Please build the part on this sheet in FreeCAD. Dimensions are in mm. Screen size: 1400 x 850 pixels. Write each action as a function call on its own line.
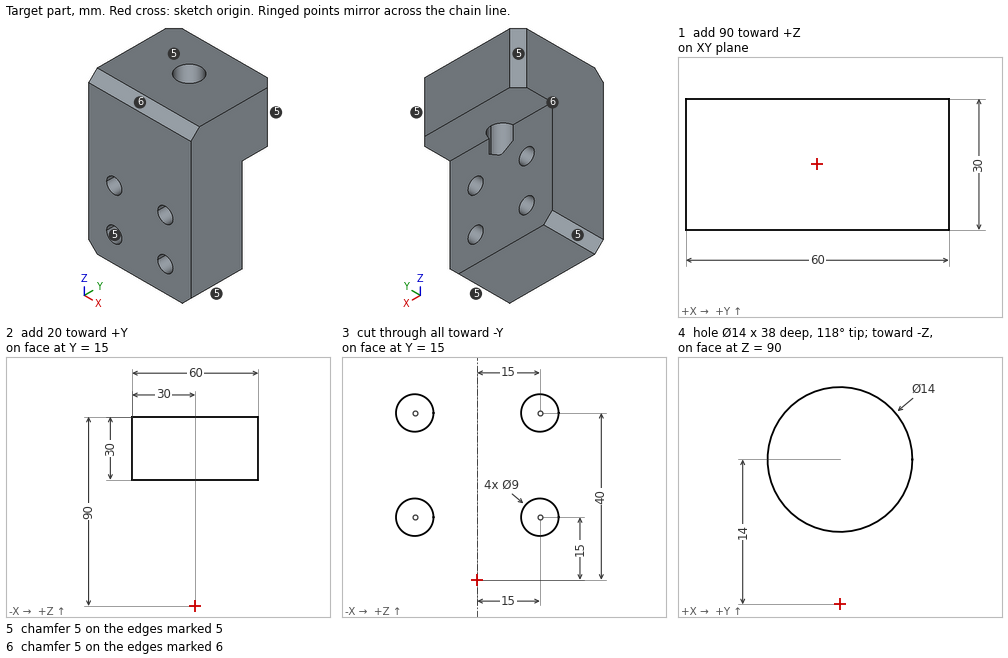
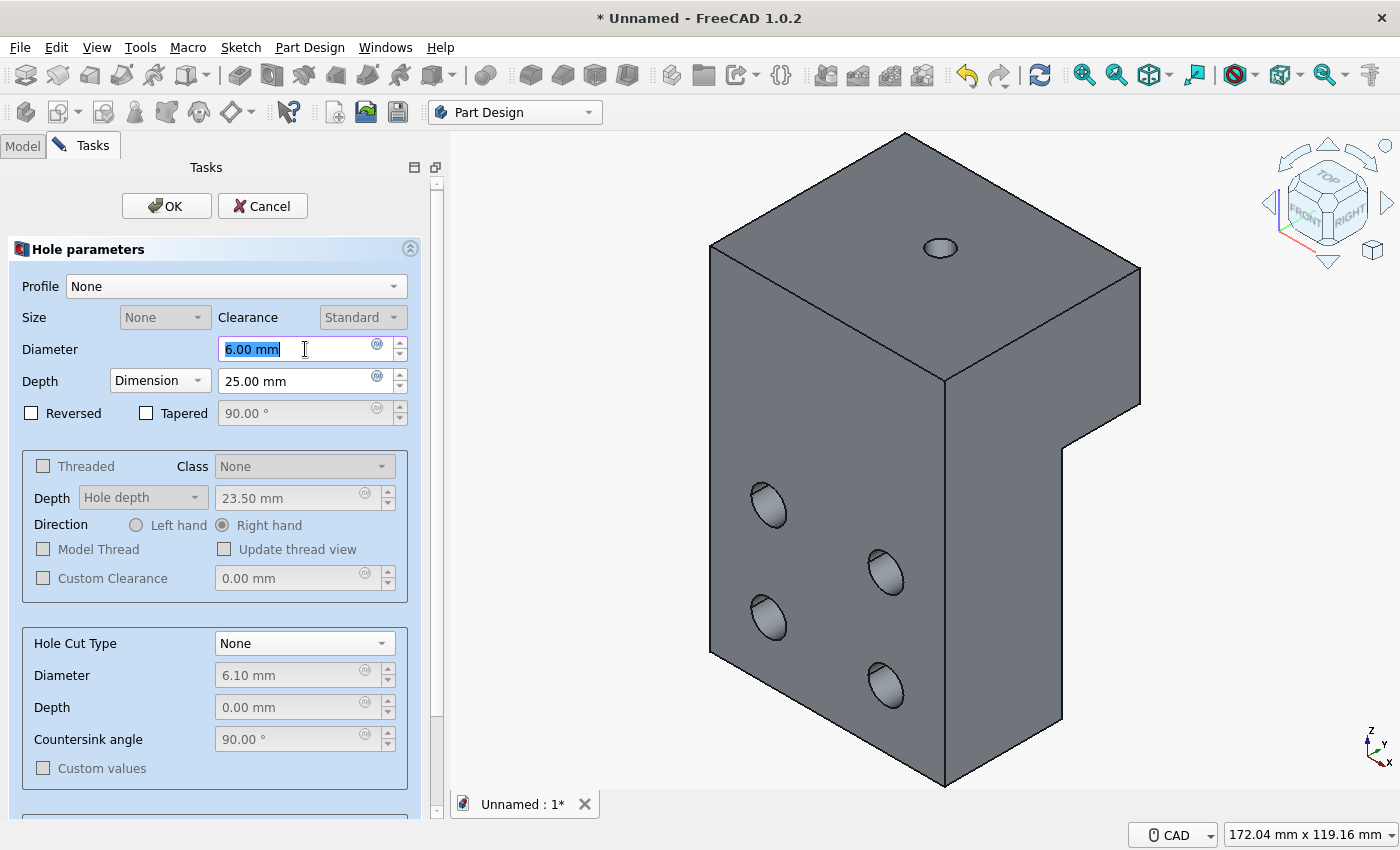
text(14)
key(Tab)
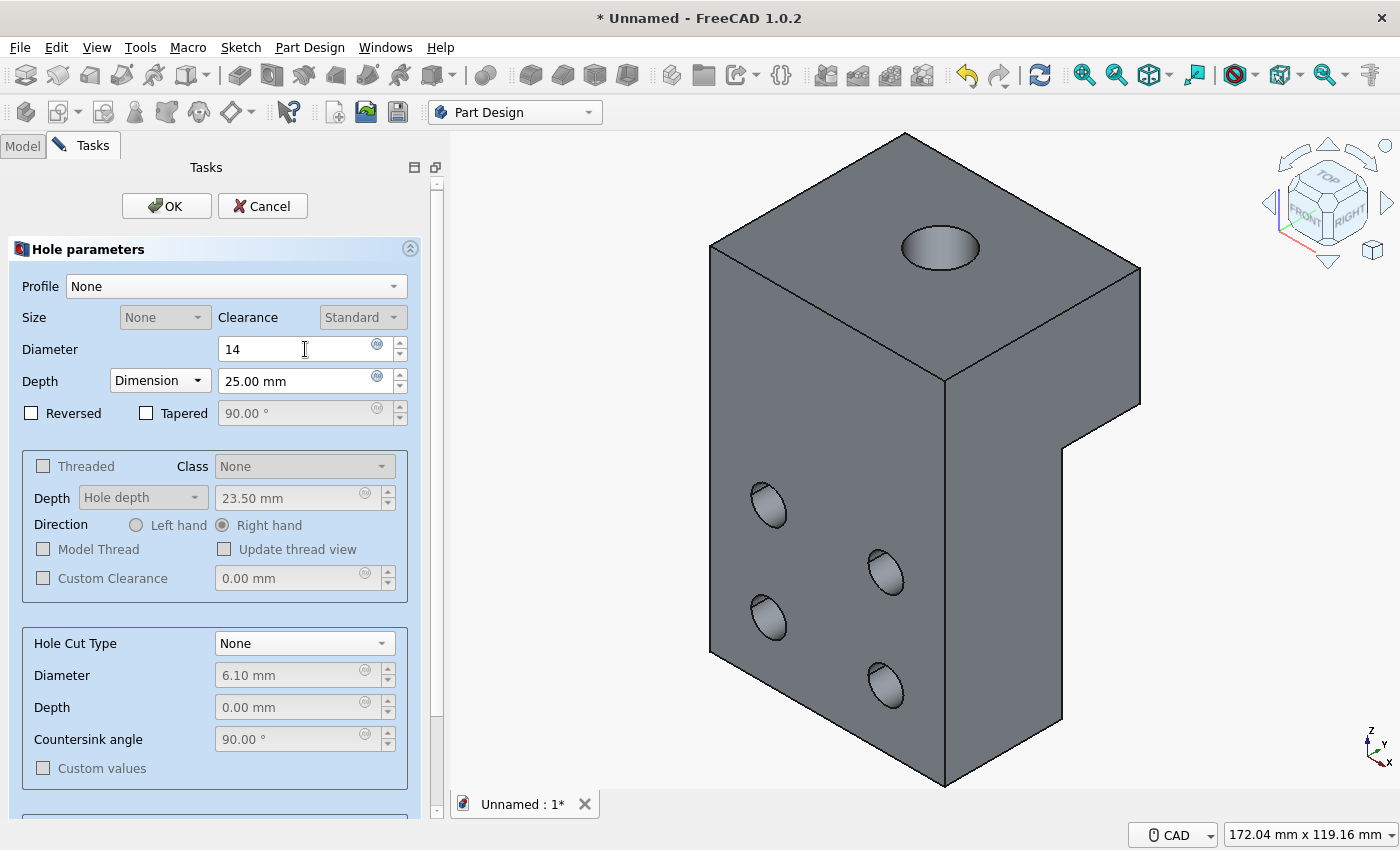
triple_click(305, 381)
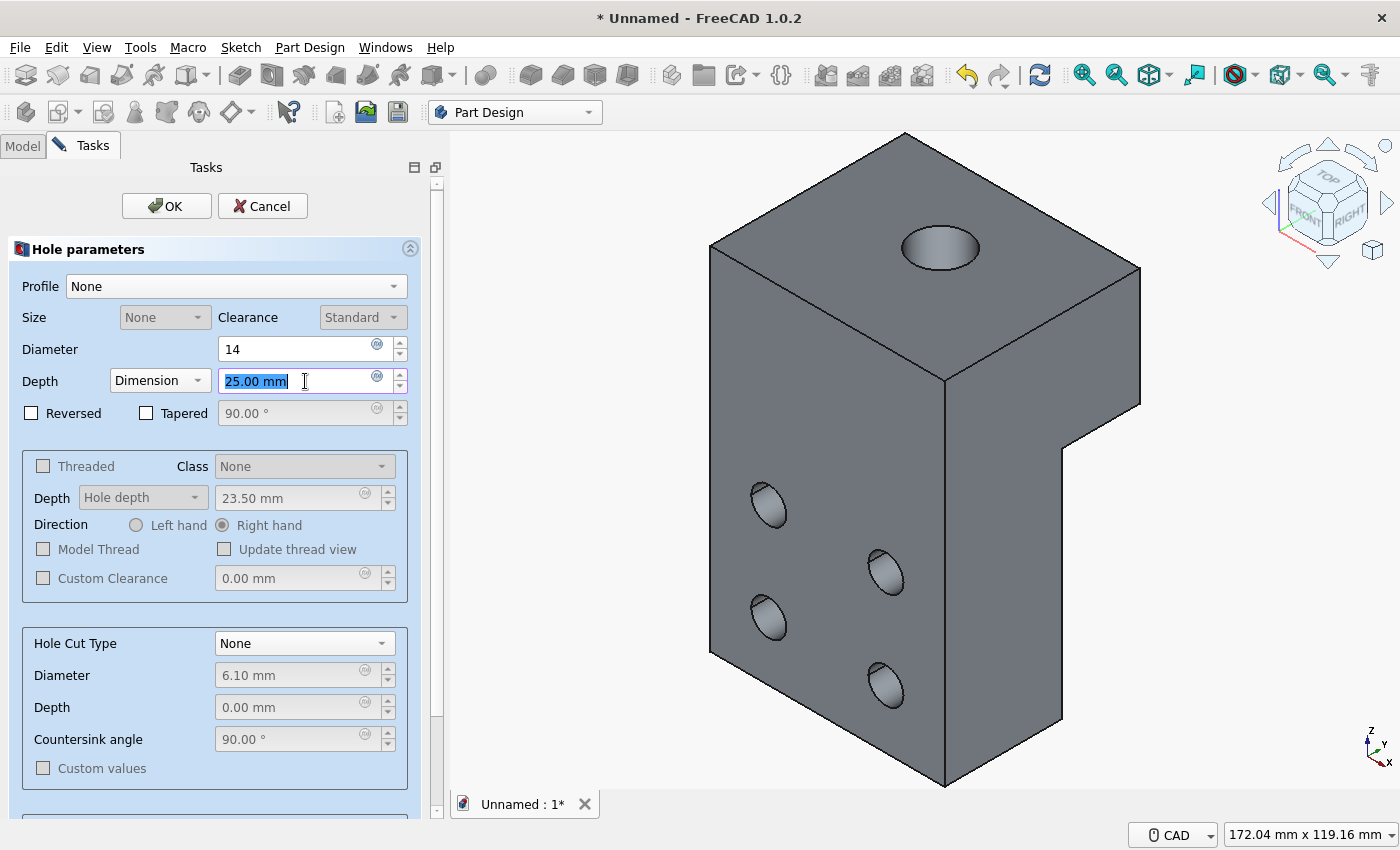
text(38)
key(Tab)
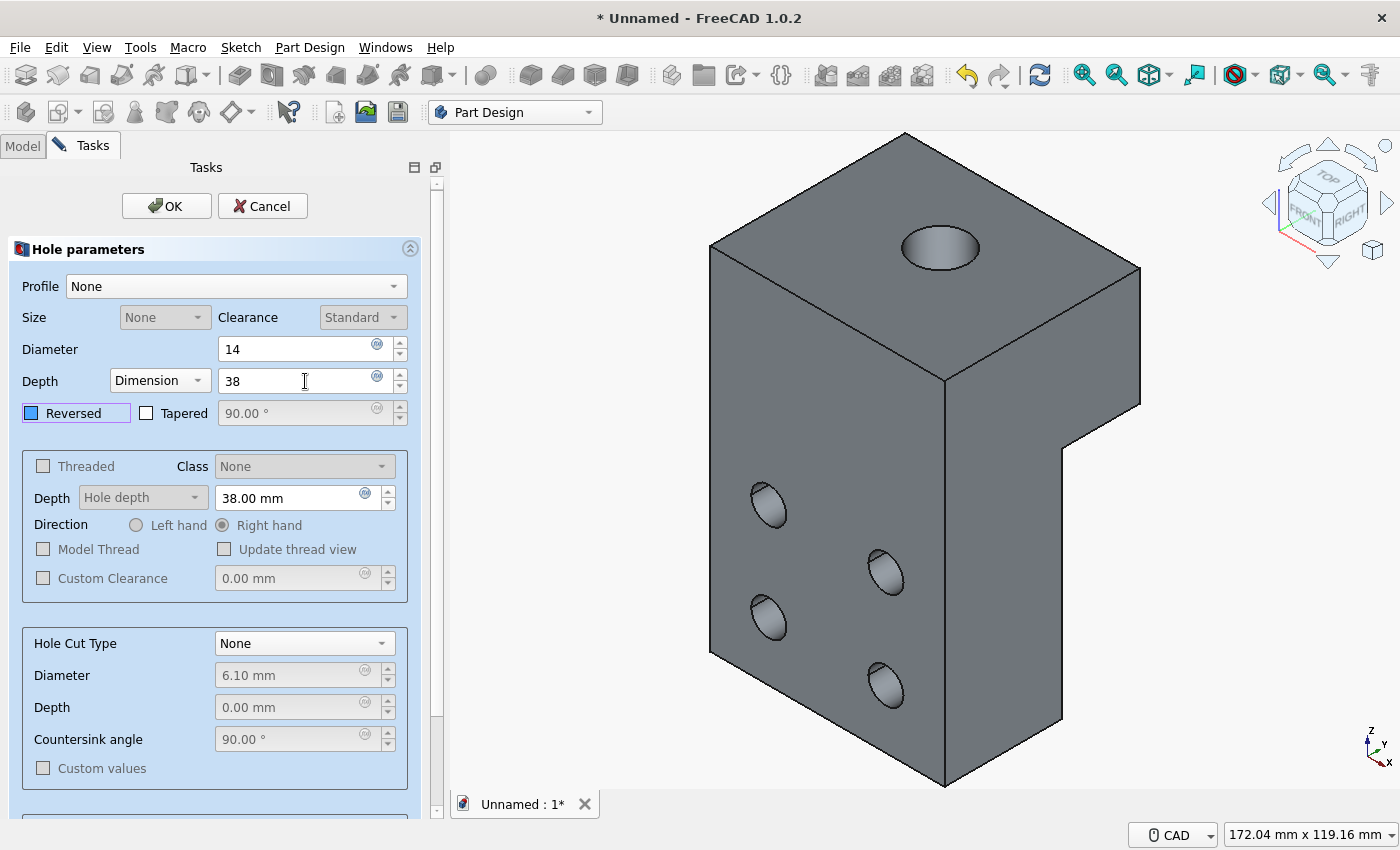
click(167, 206)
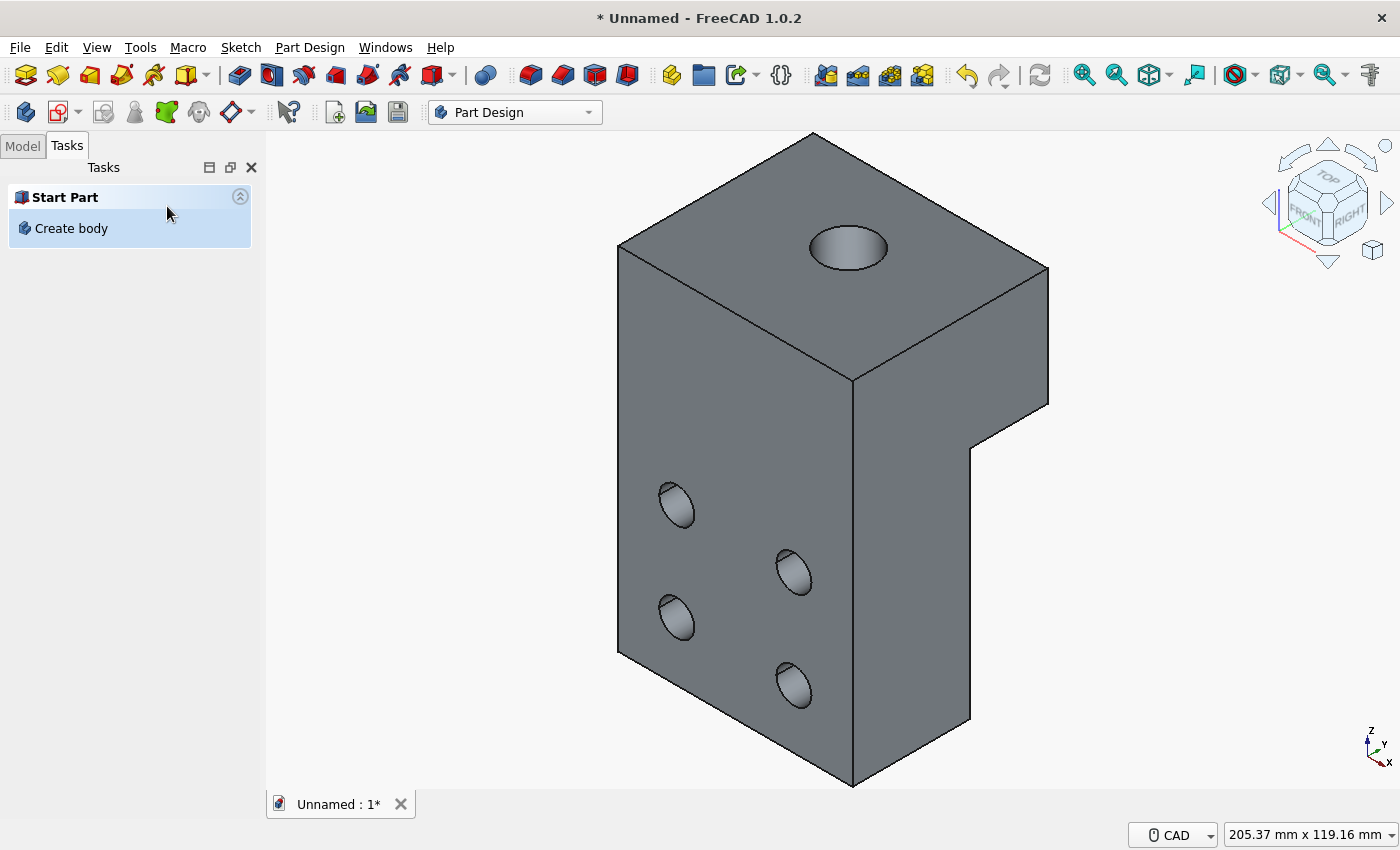
key(2)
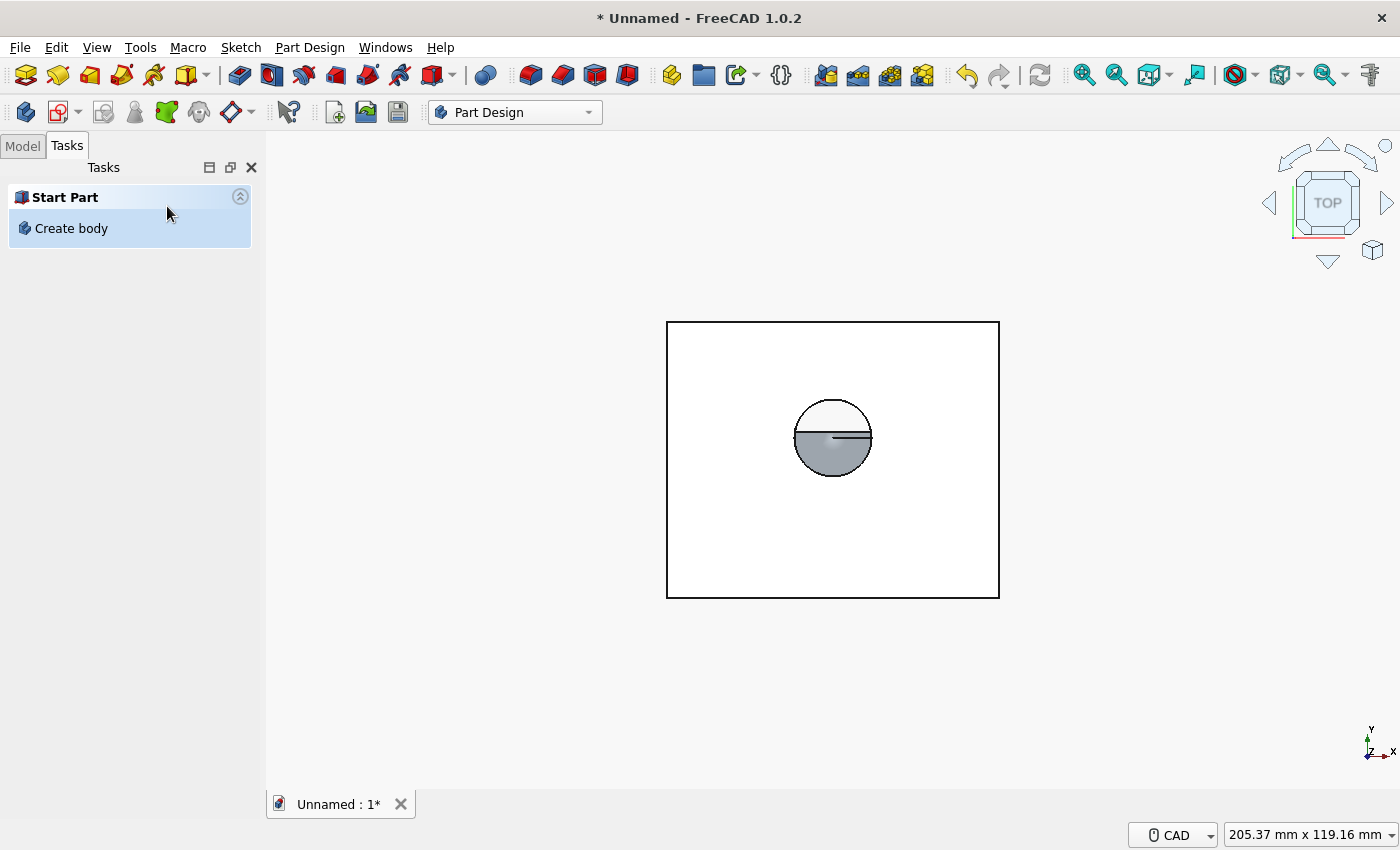
click(1086, 76)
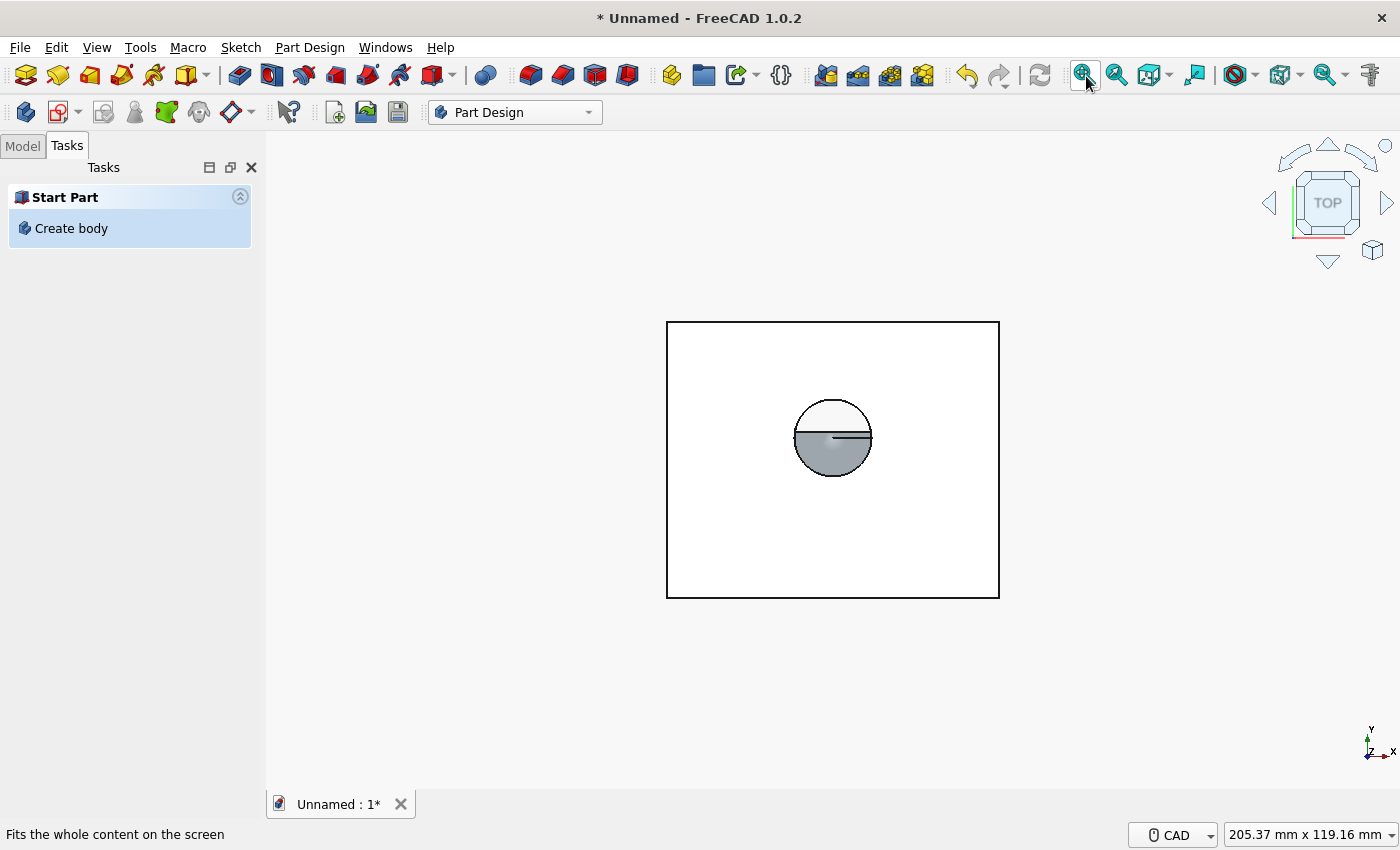
key(0)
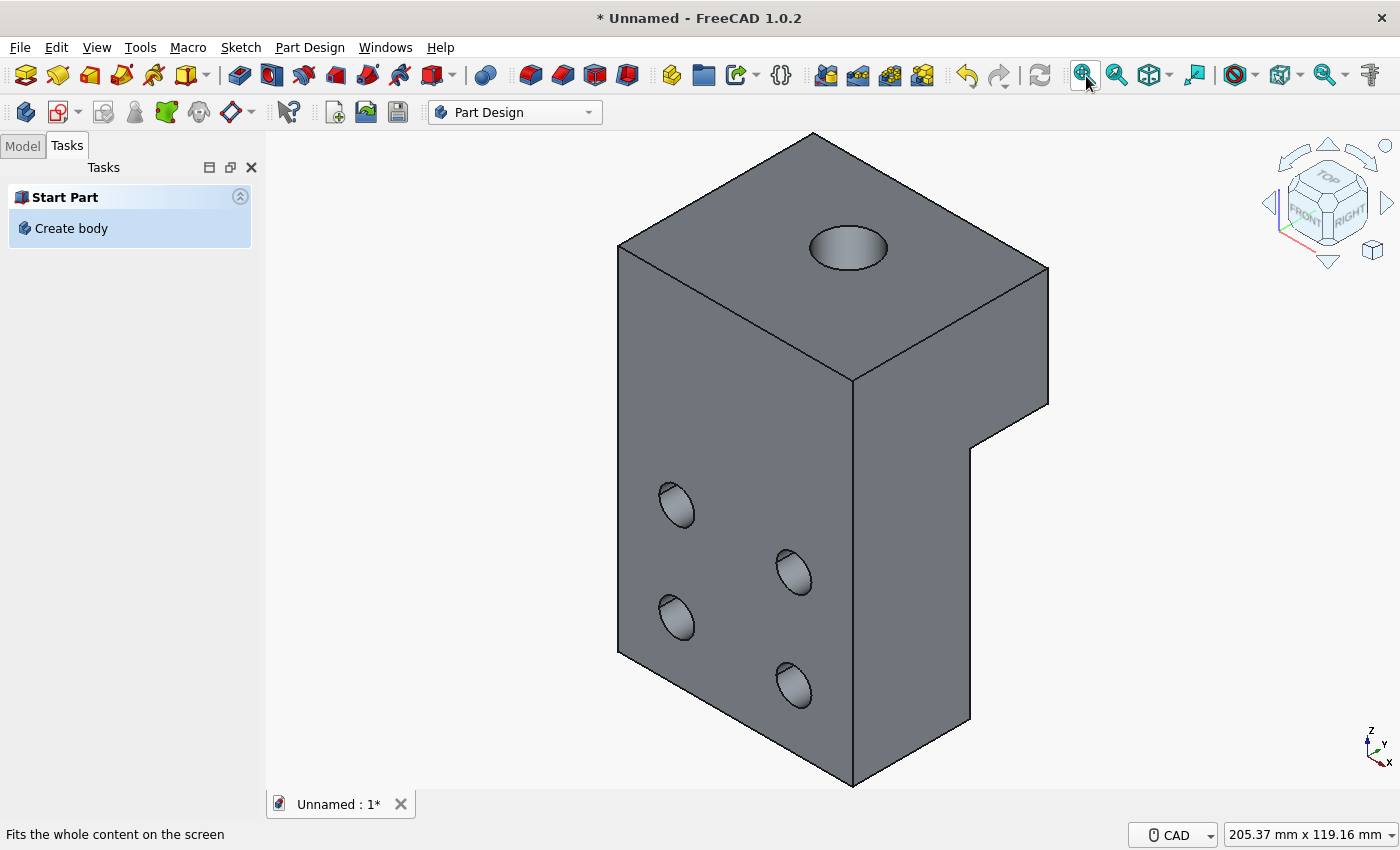
key(1)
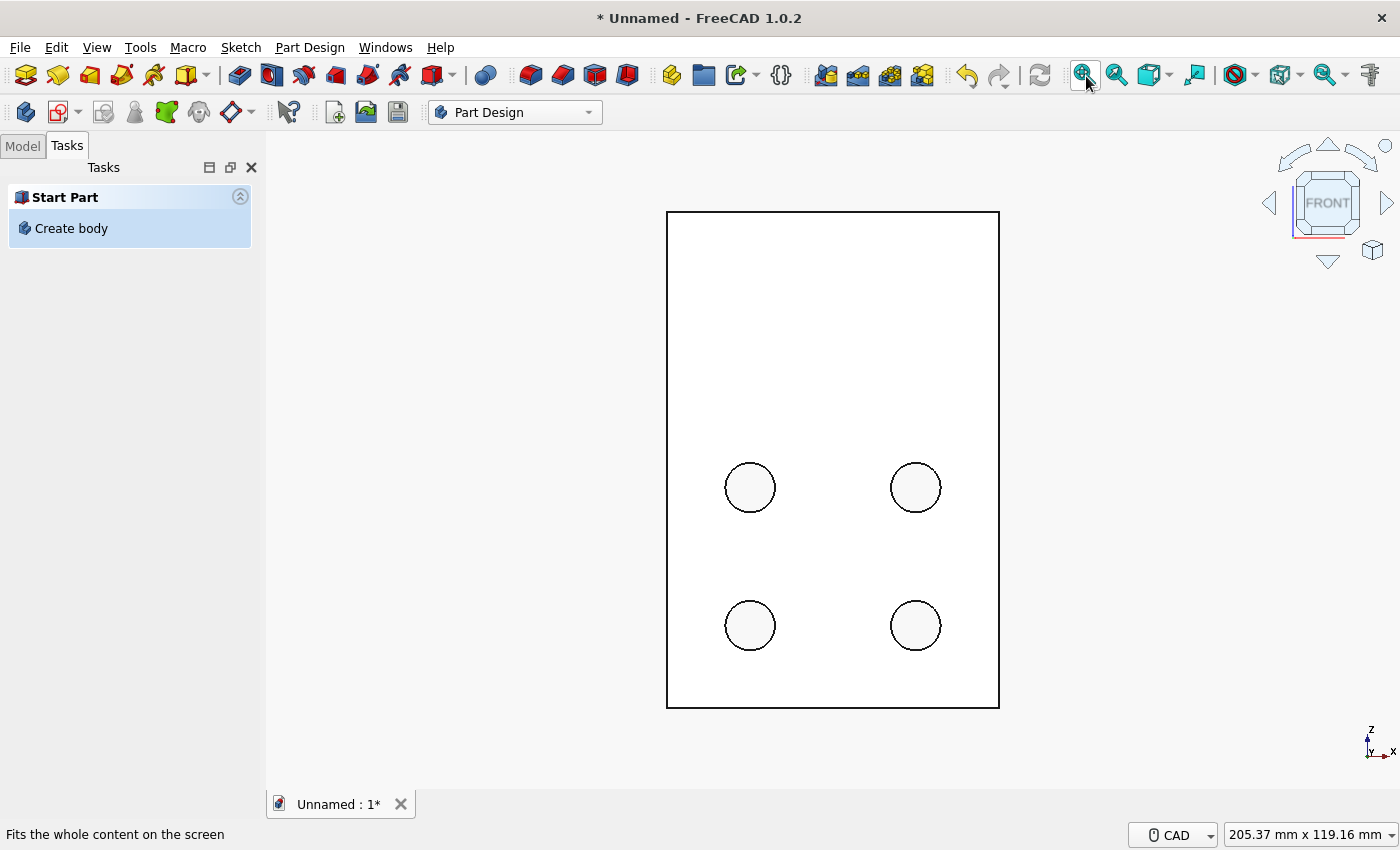
key(3)